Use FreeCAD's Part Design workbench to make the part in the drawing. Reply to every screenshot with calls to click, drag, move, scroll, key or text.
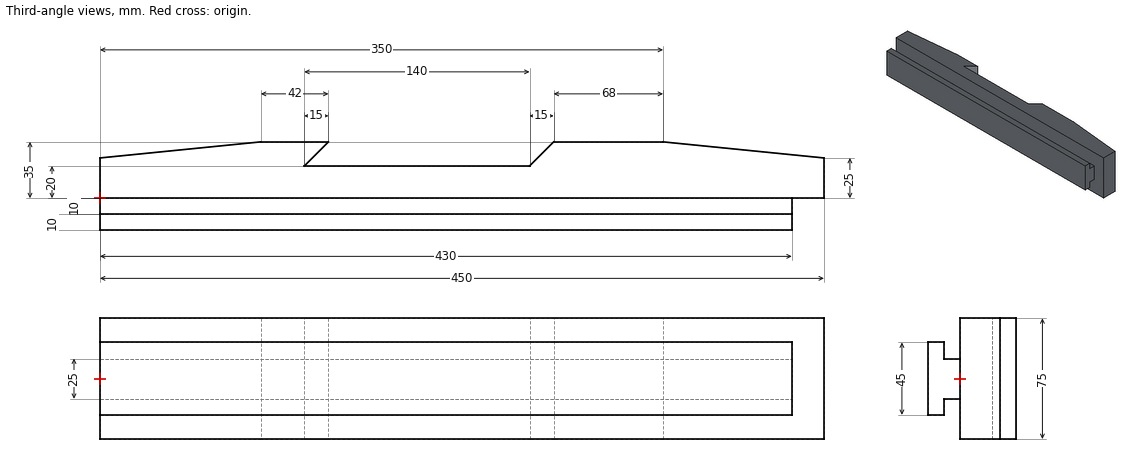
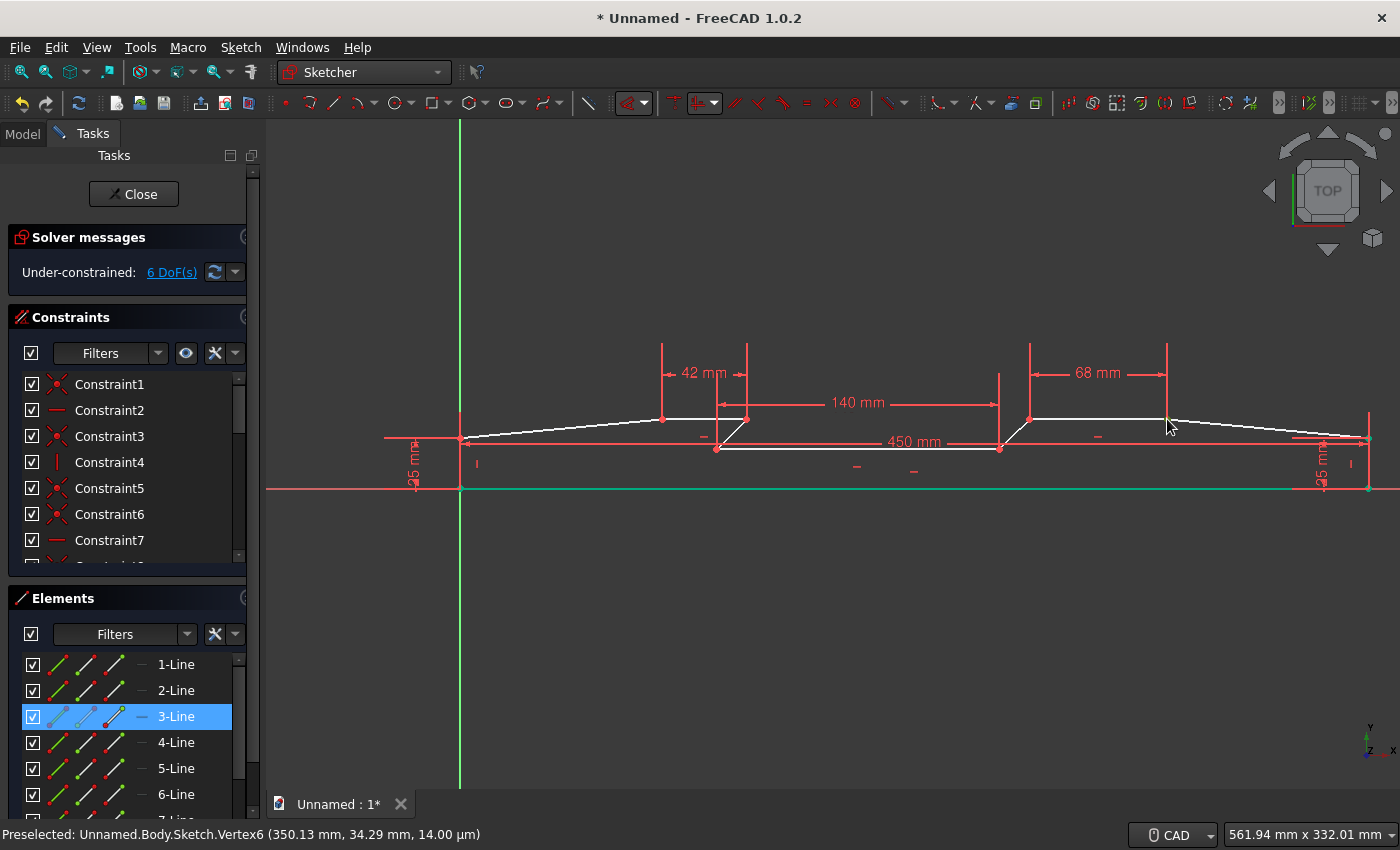
key(i)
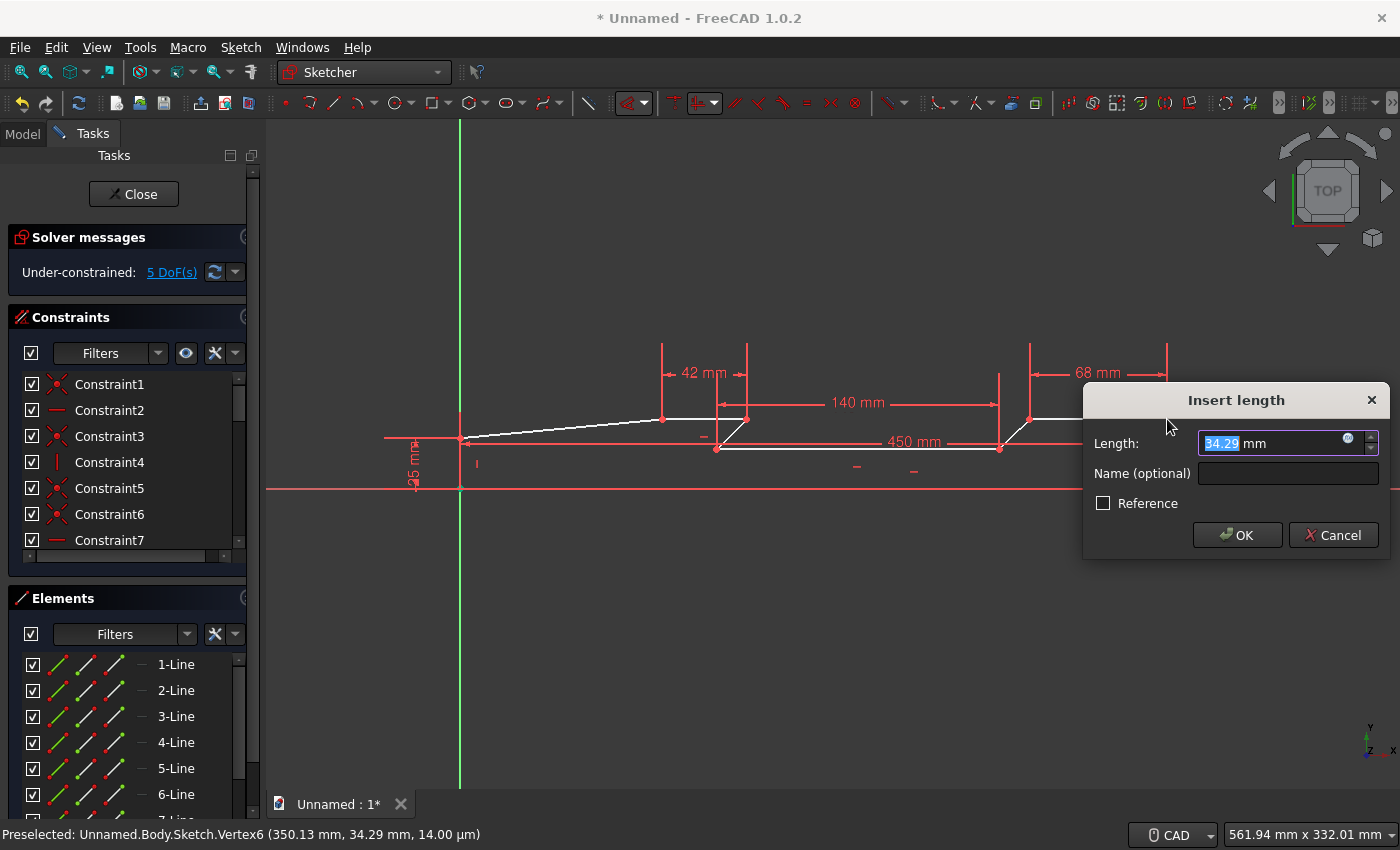
text(35)
key(Return)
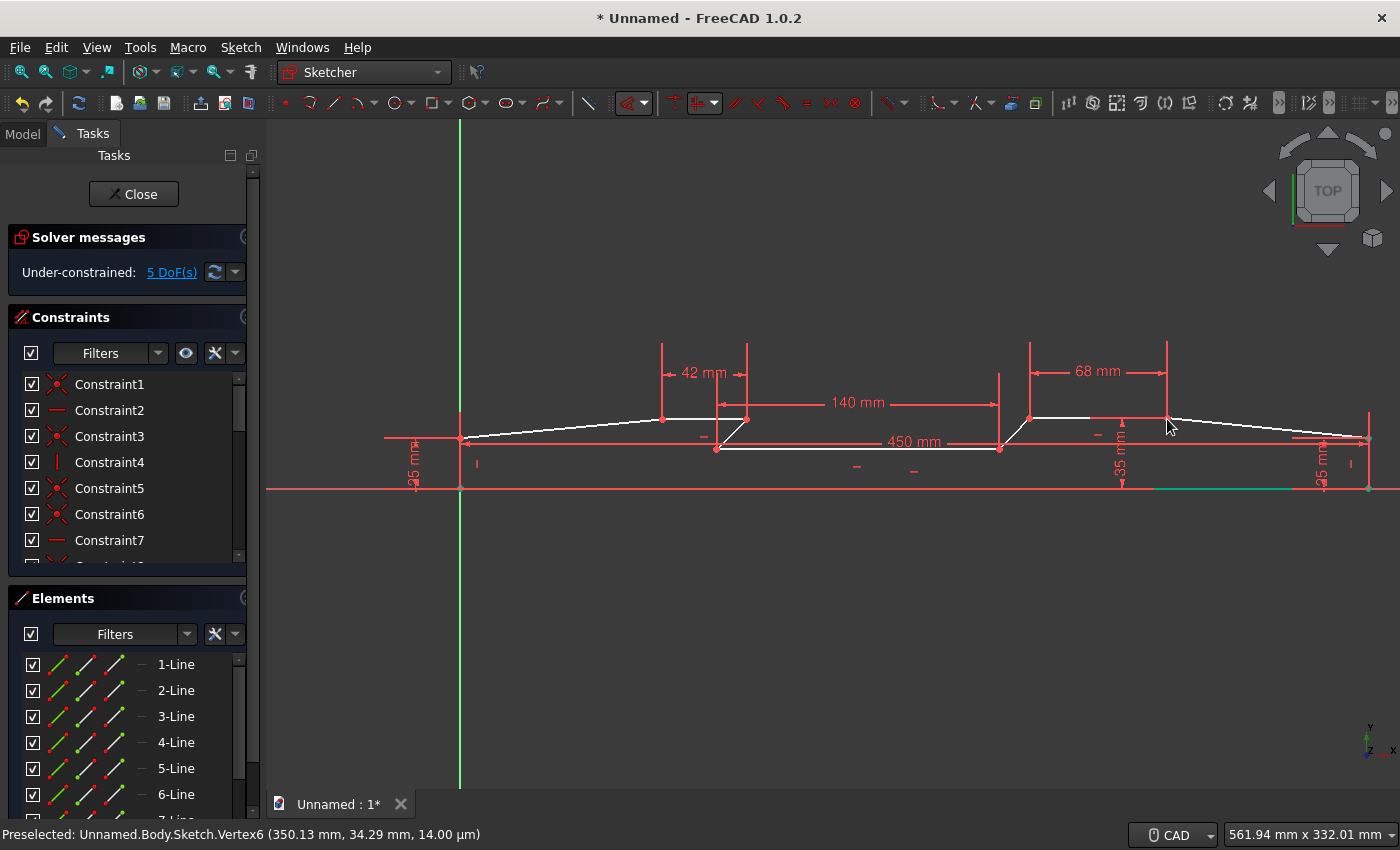
click(999, 449)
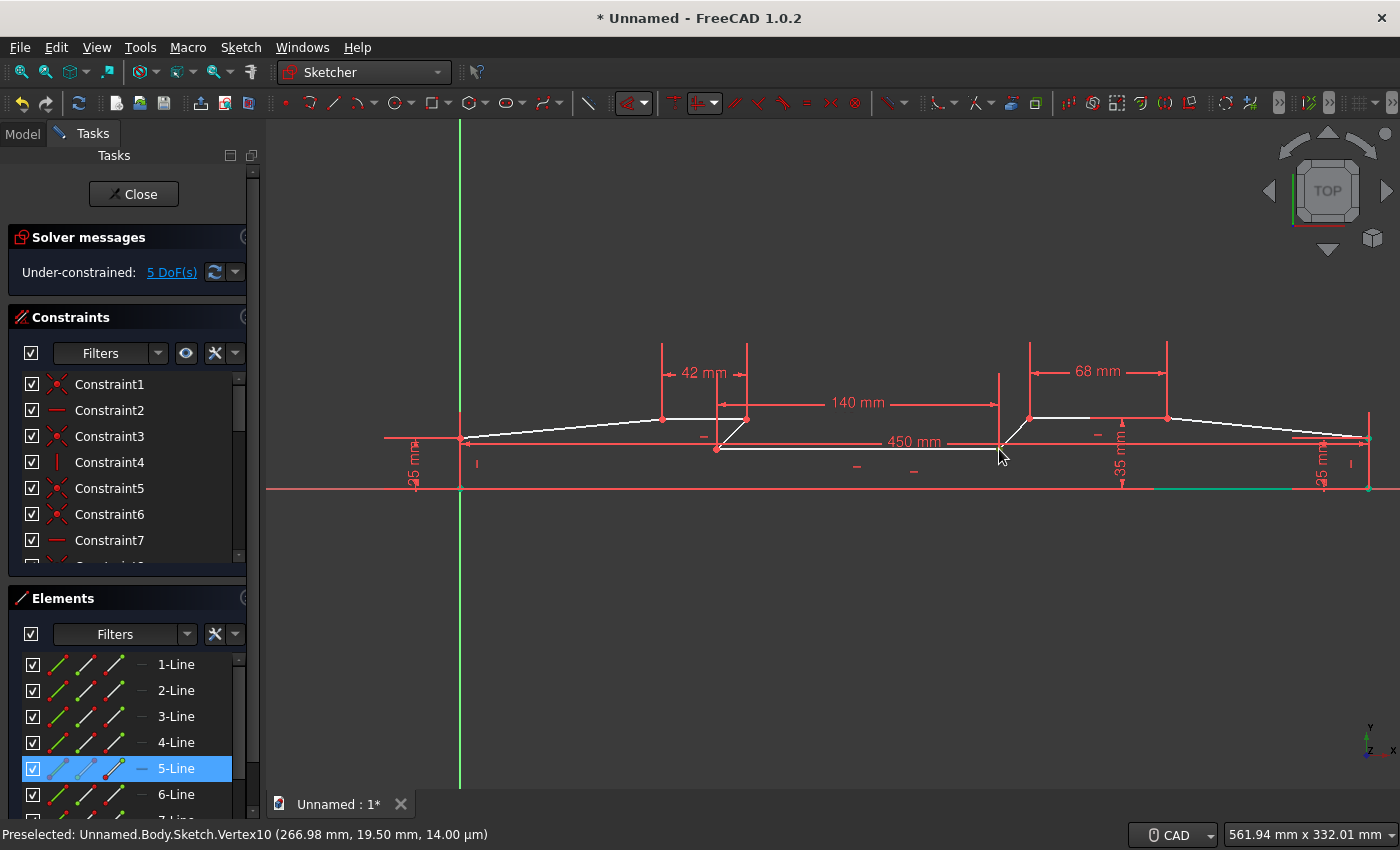
click(646, 104)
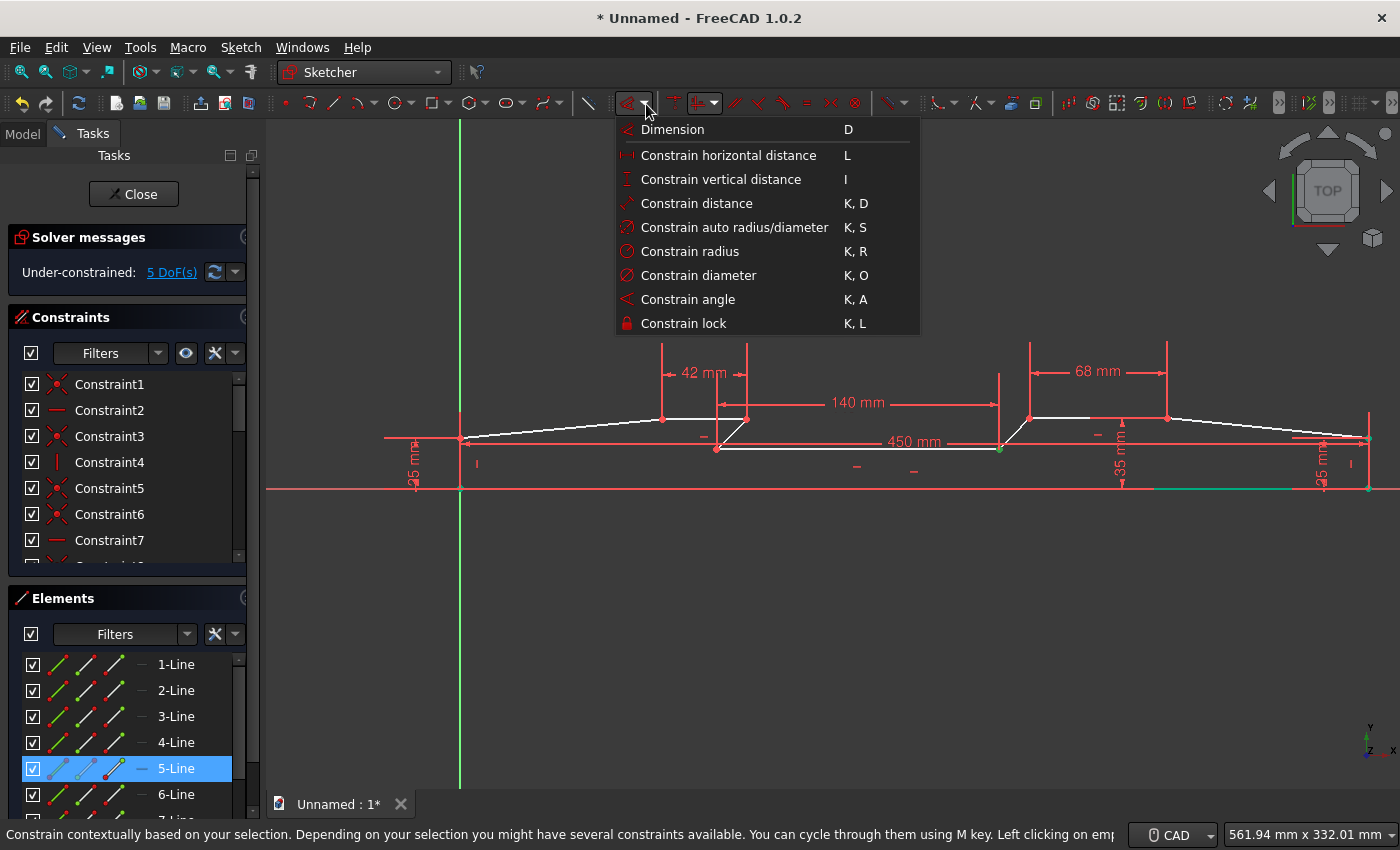
click(768, 179)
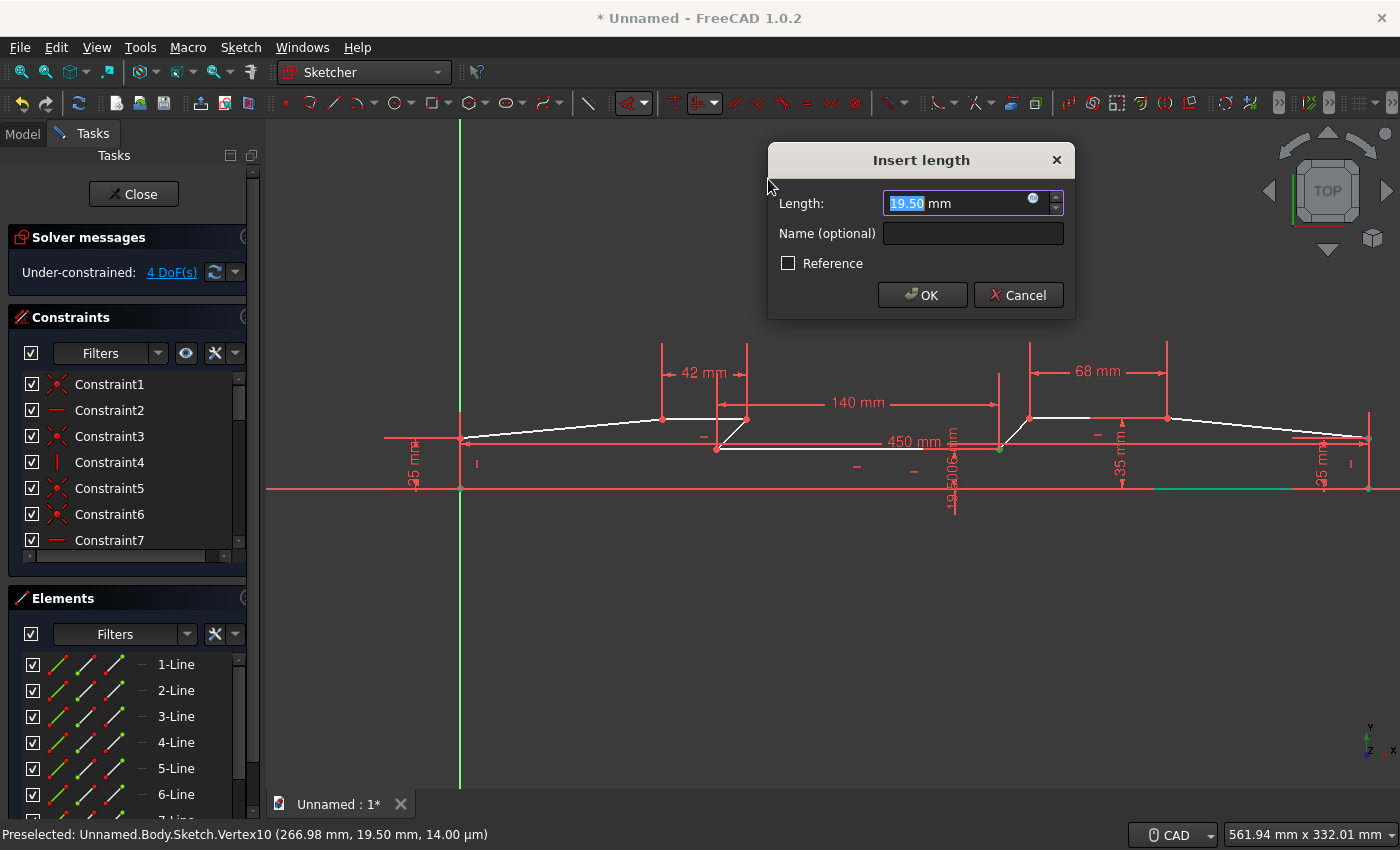
text(20)
key(Return)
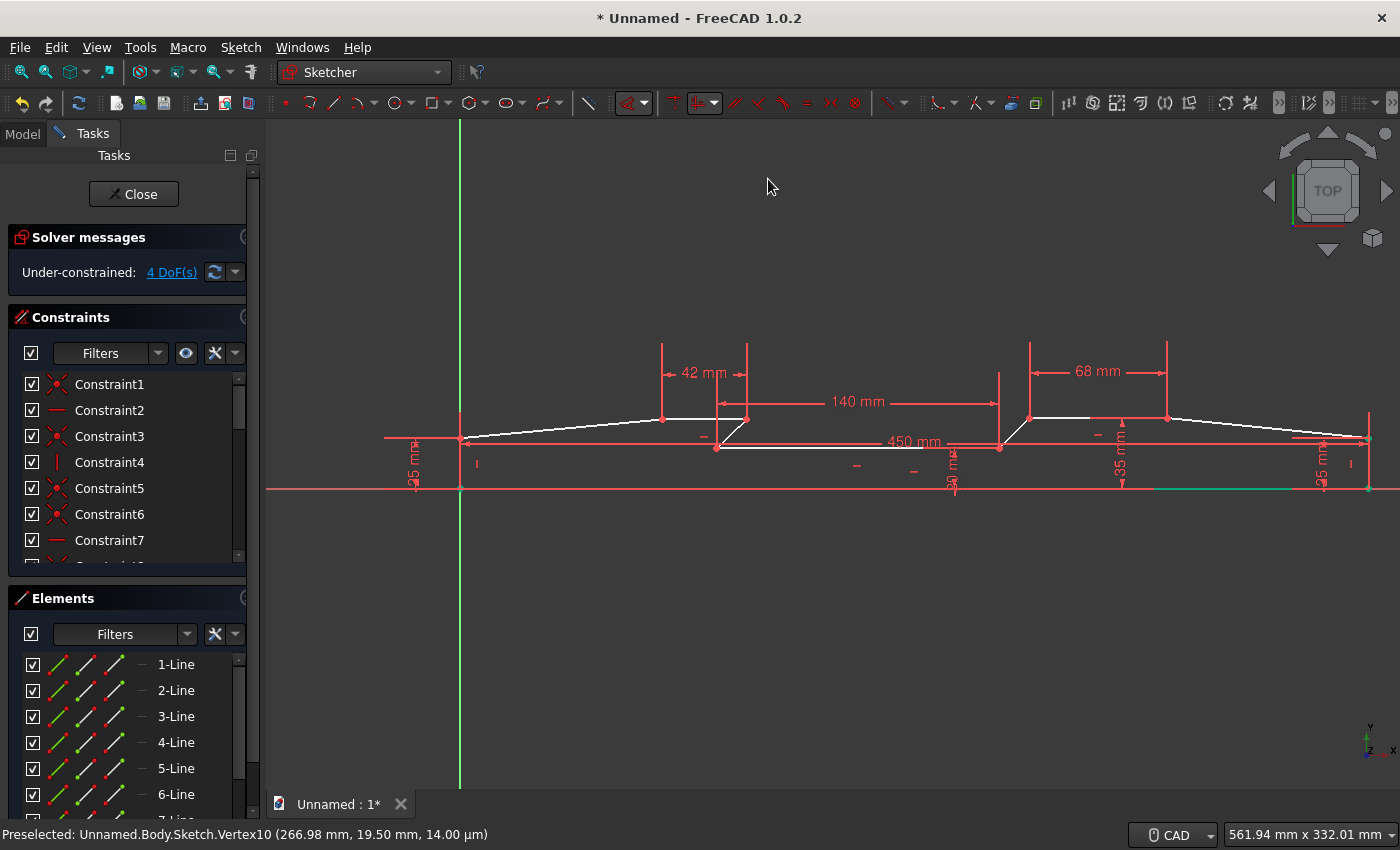
click(747, 419)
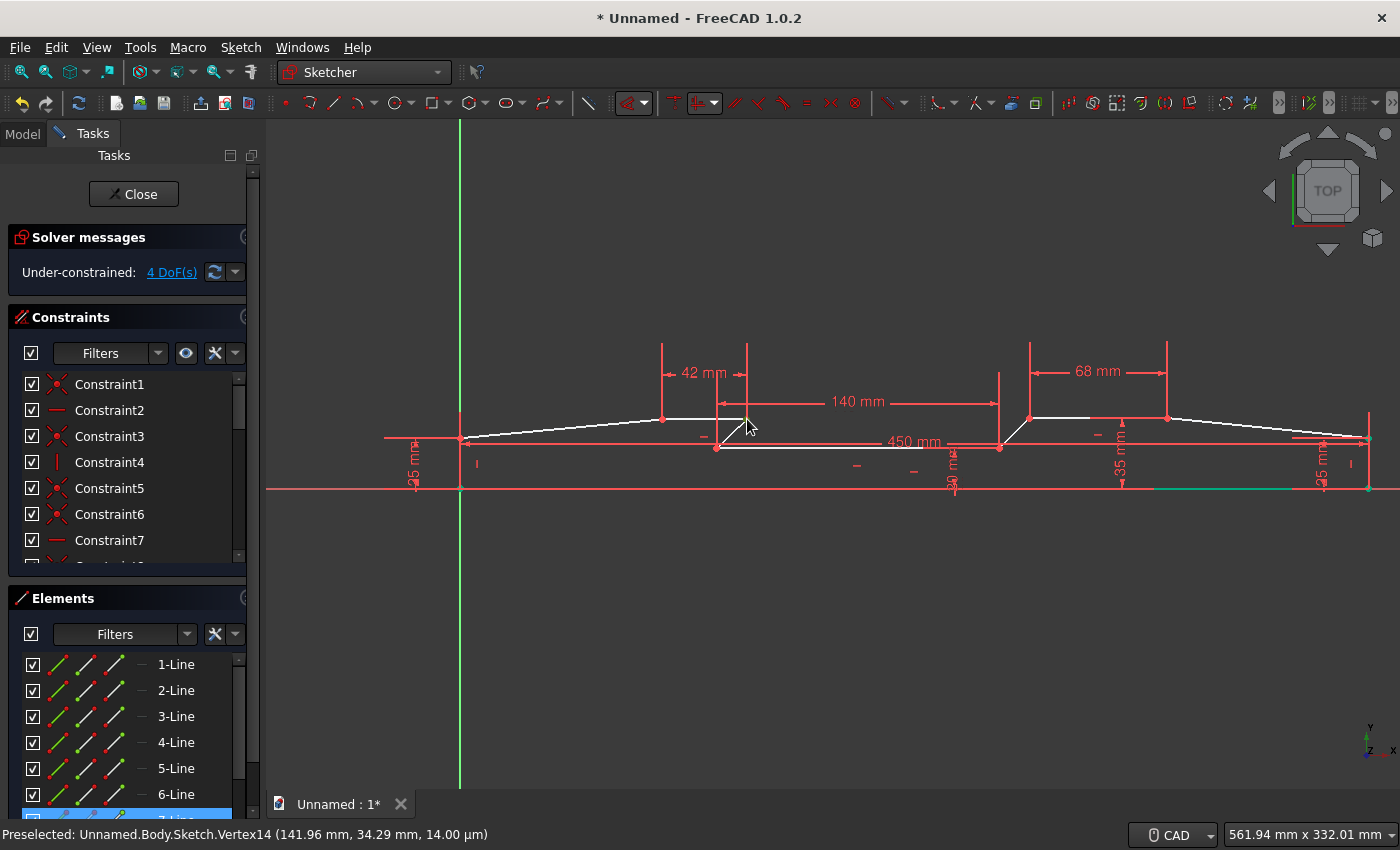
click(646, 104)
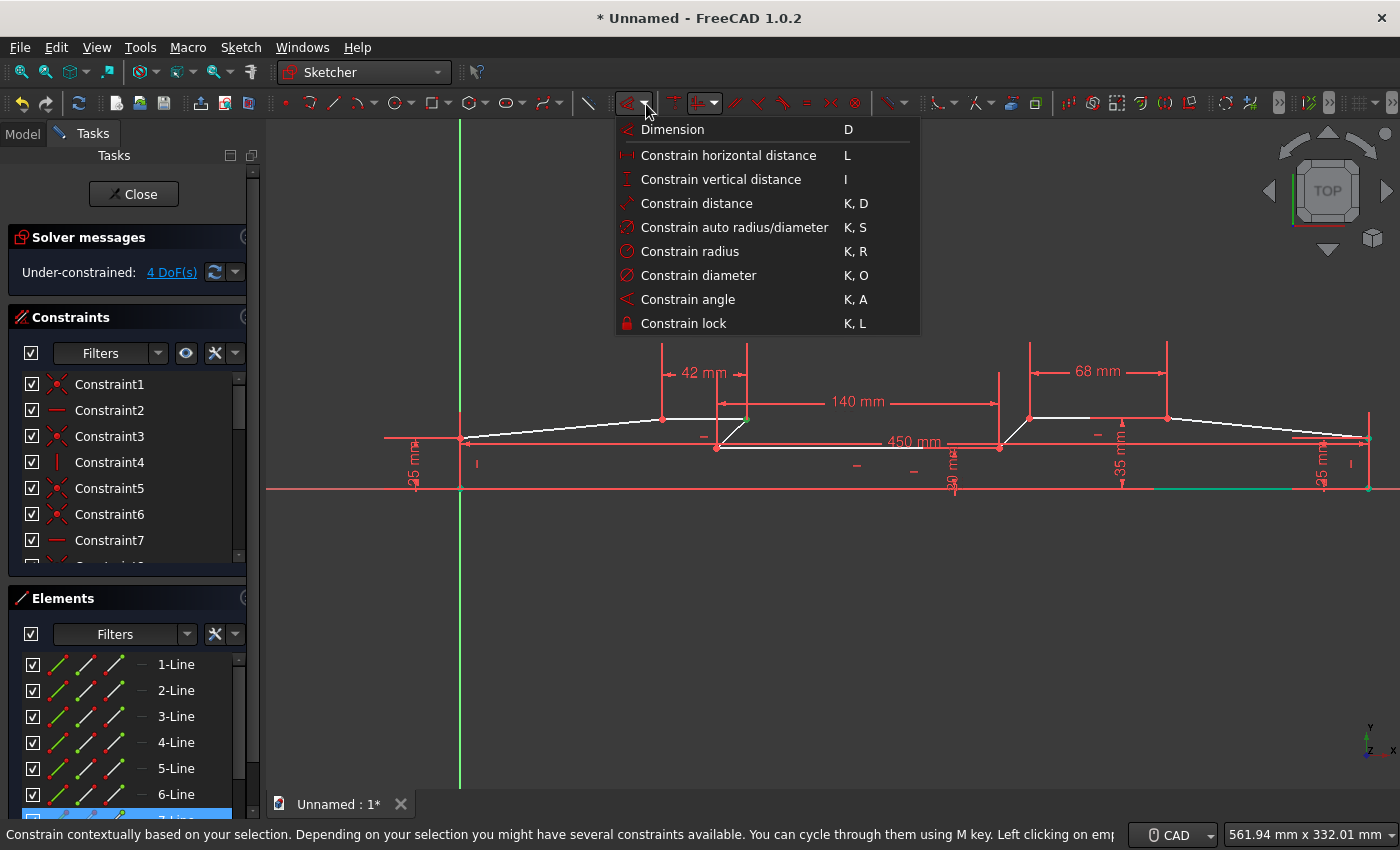
click(768, 179)